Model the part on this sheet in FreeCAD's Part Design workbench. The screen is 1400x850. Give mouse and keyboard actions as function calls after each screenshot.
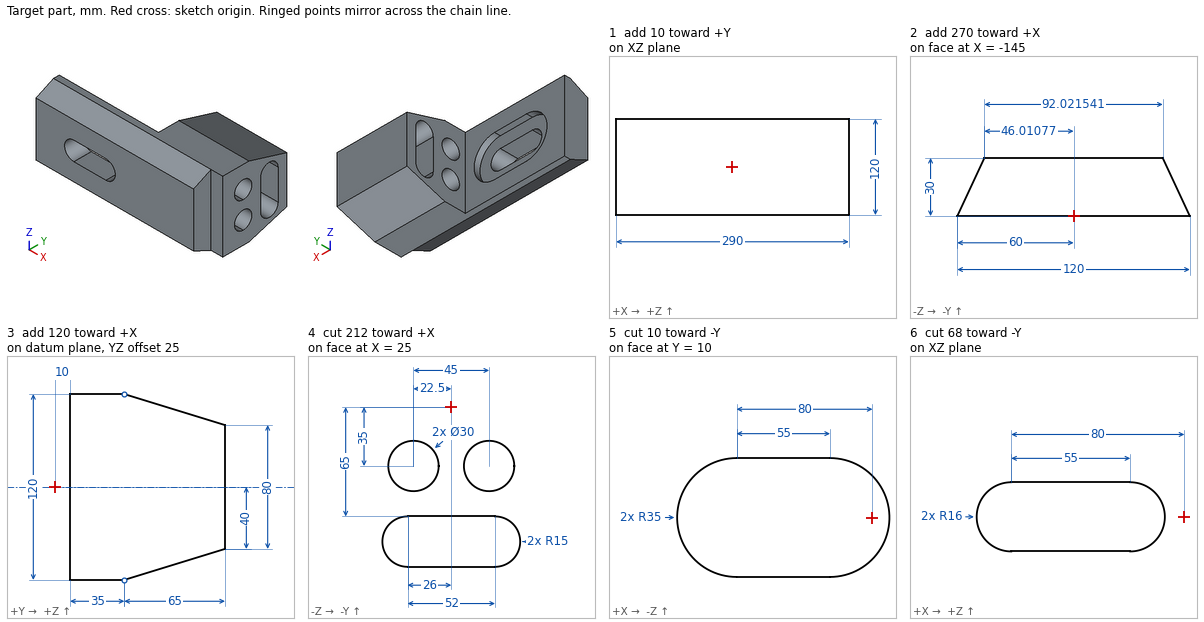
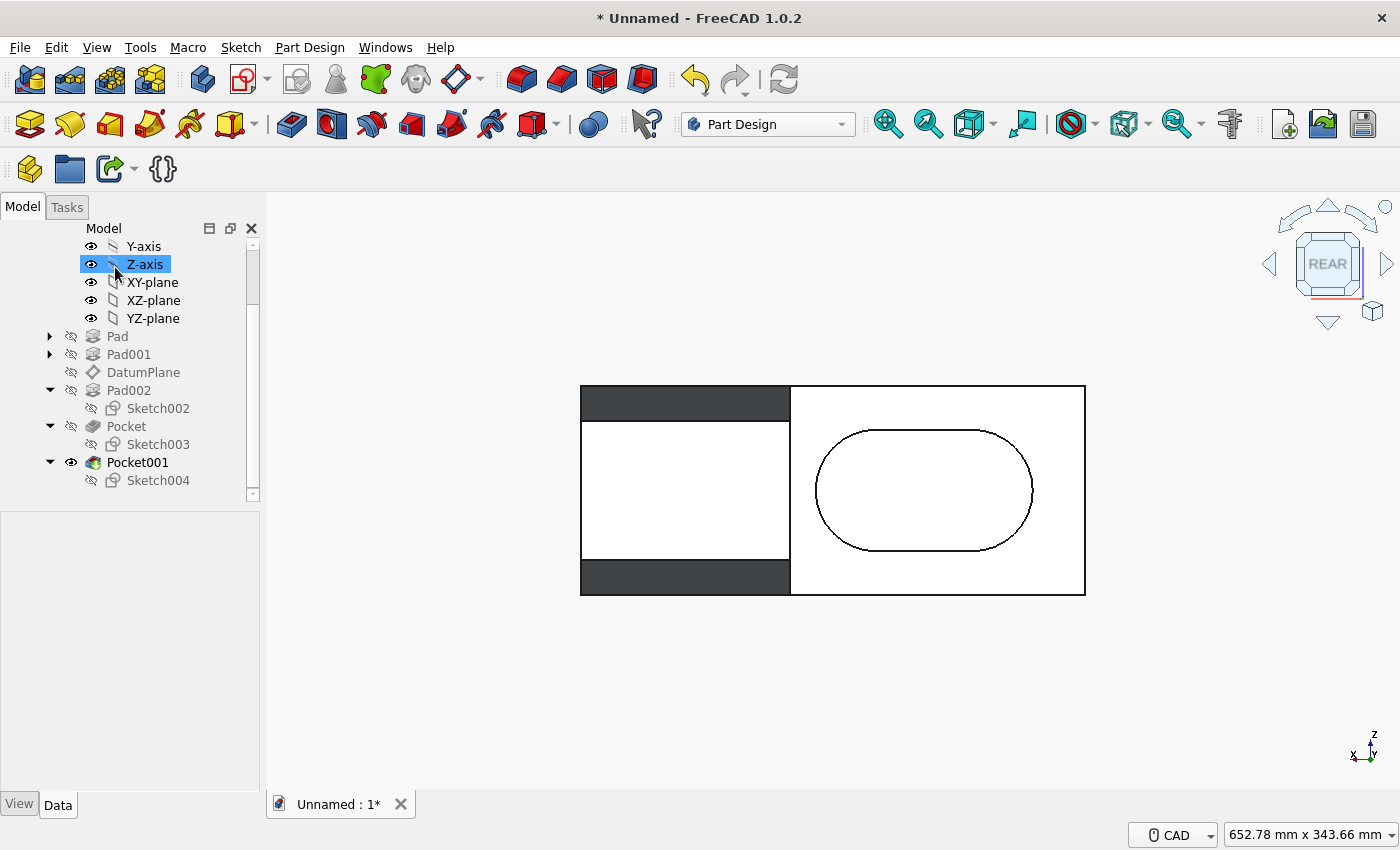
key(v)
key(f)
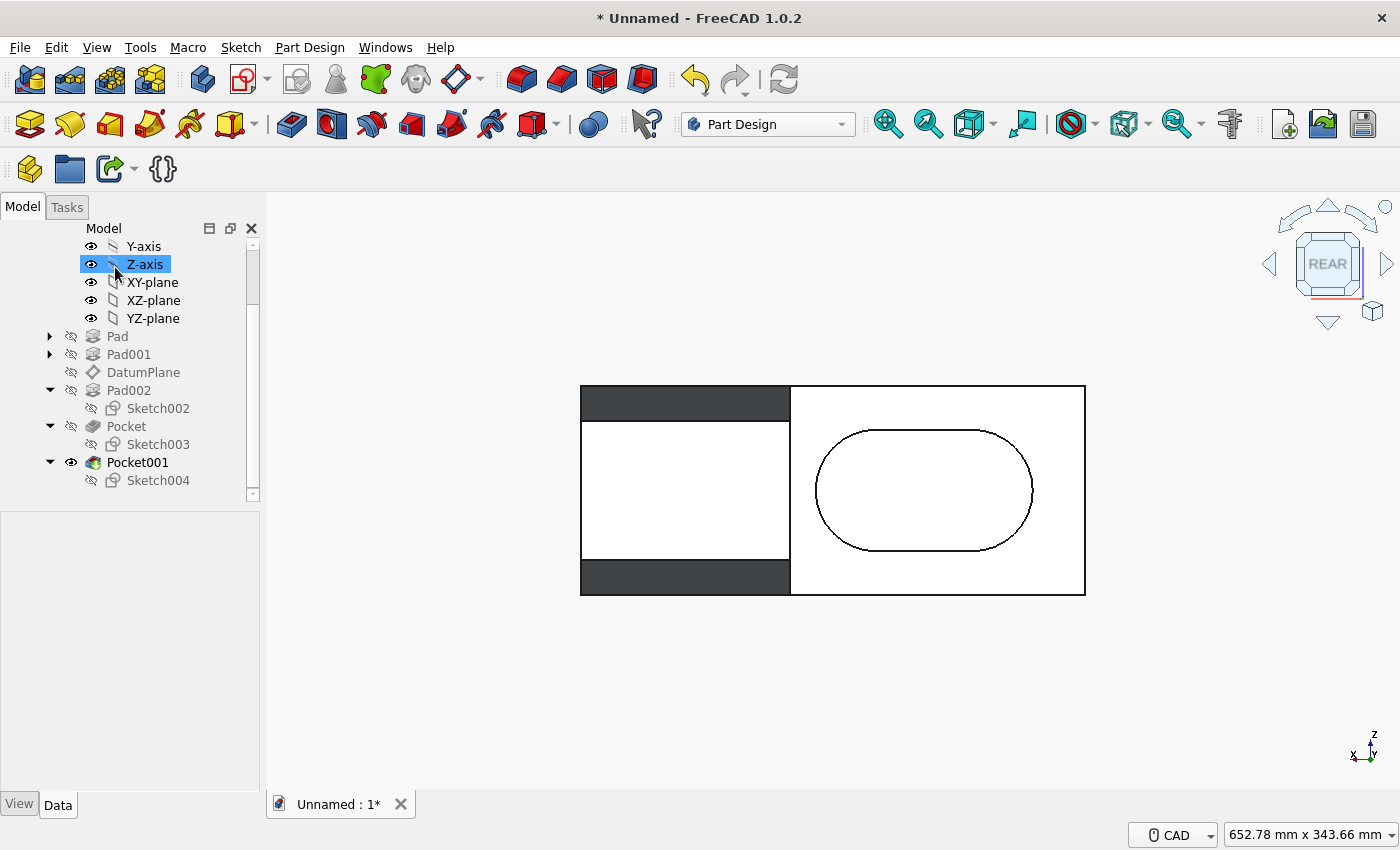
click(244, 80)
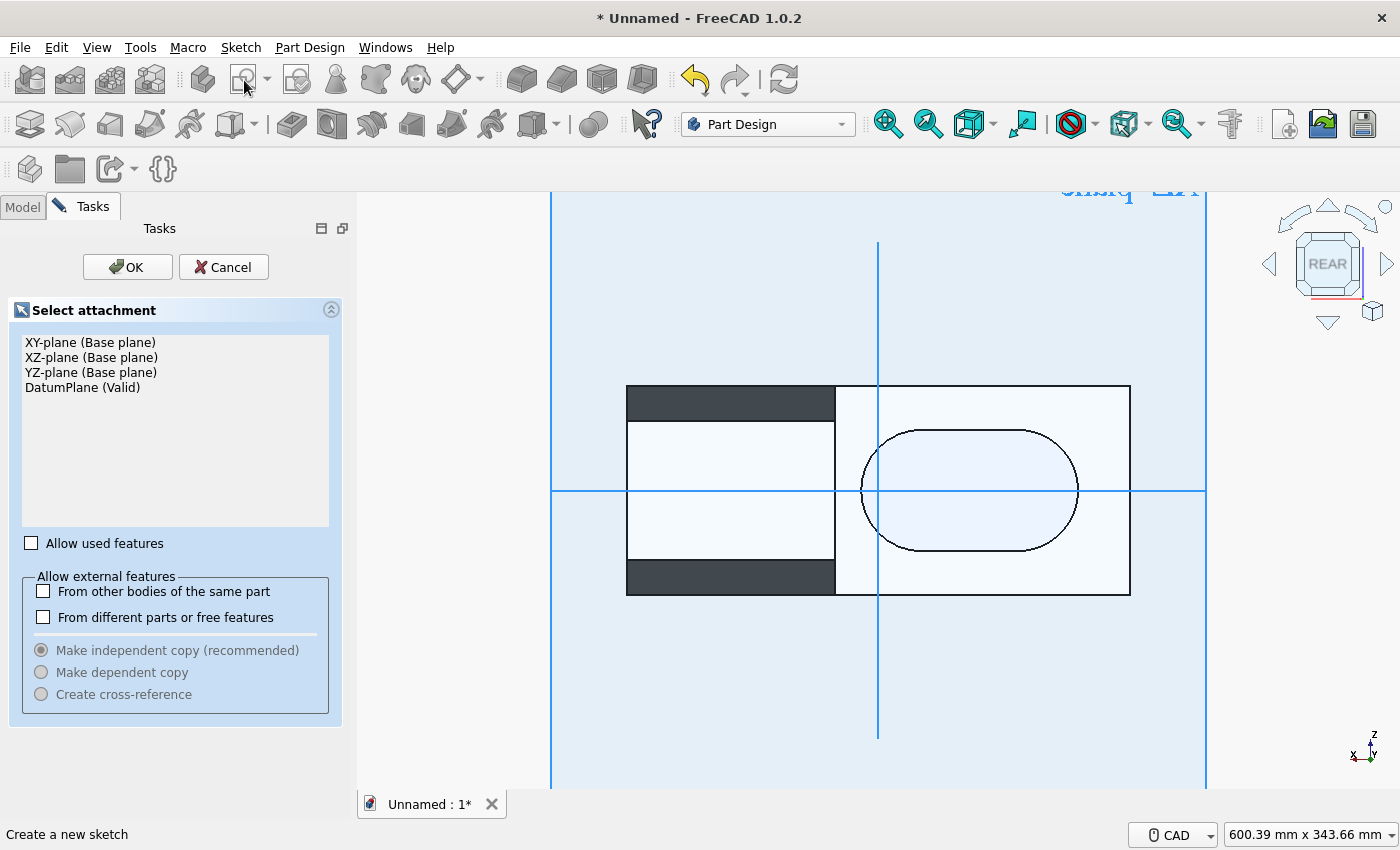
click(82, 358)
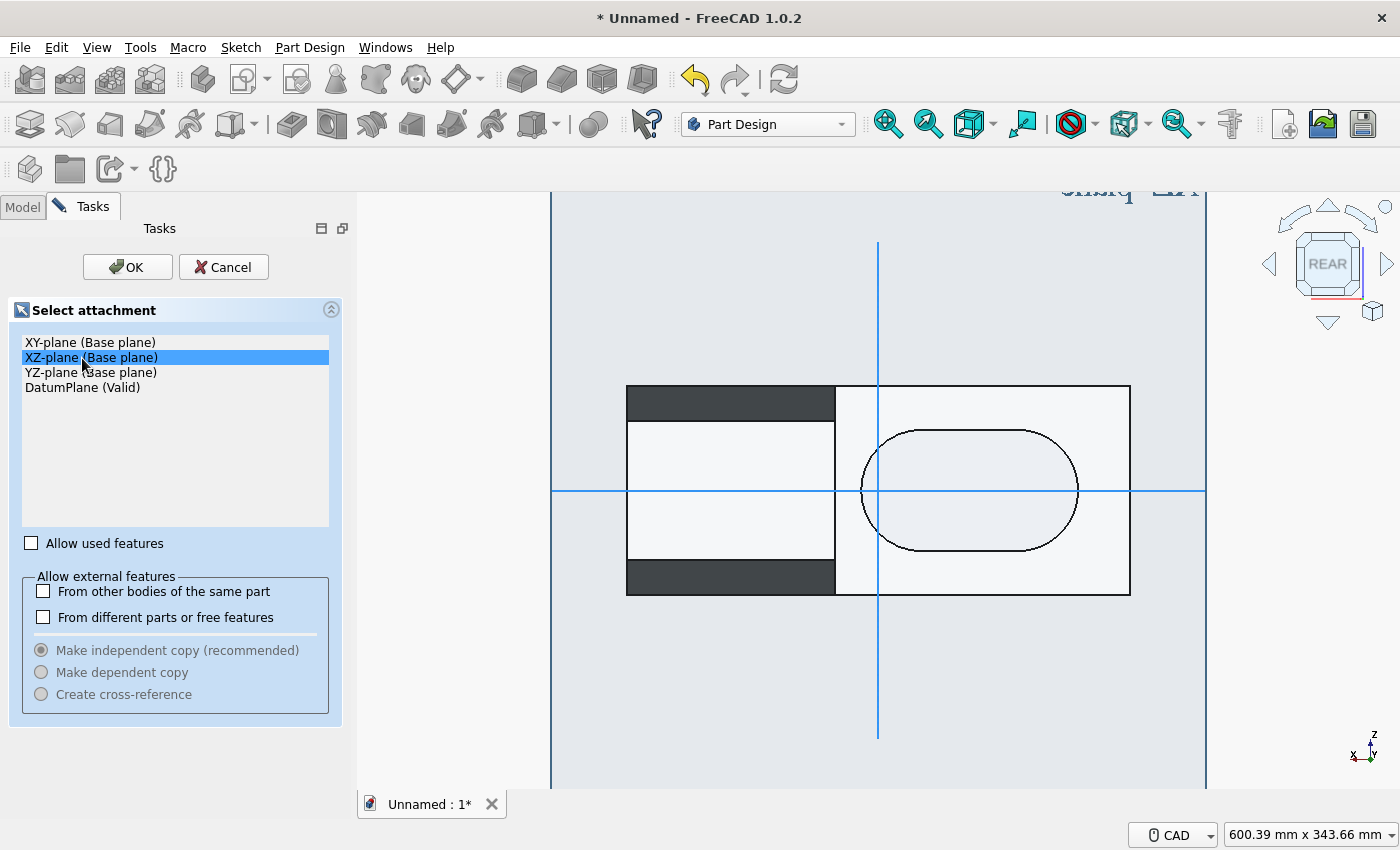
click(128, 267)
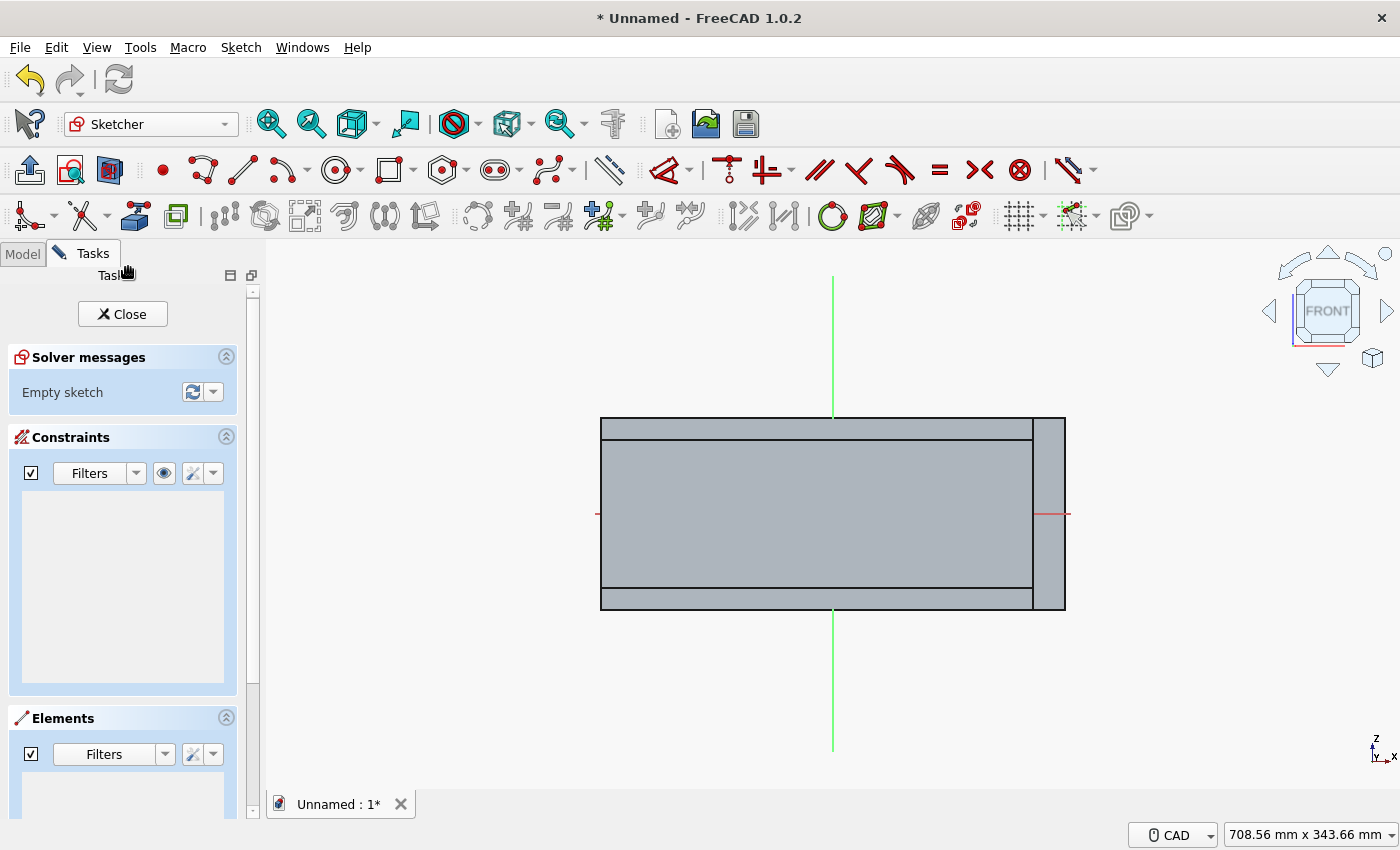
key(q)
key(s)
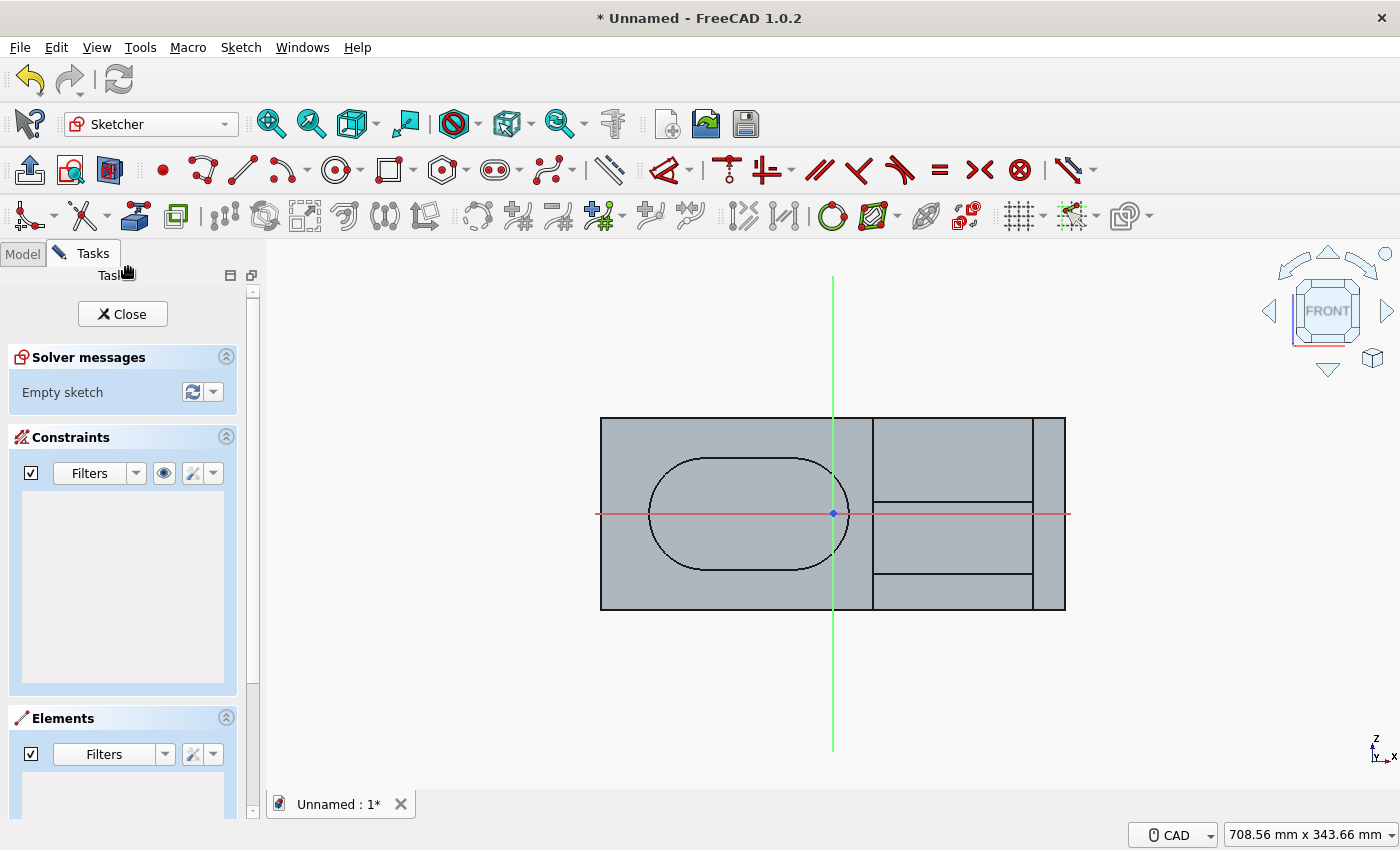
scroll(753, 514, up, 7)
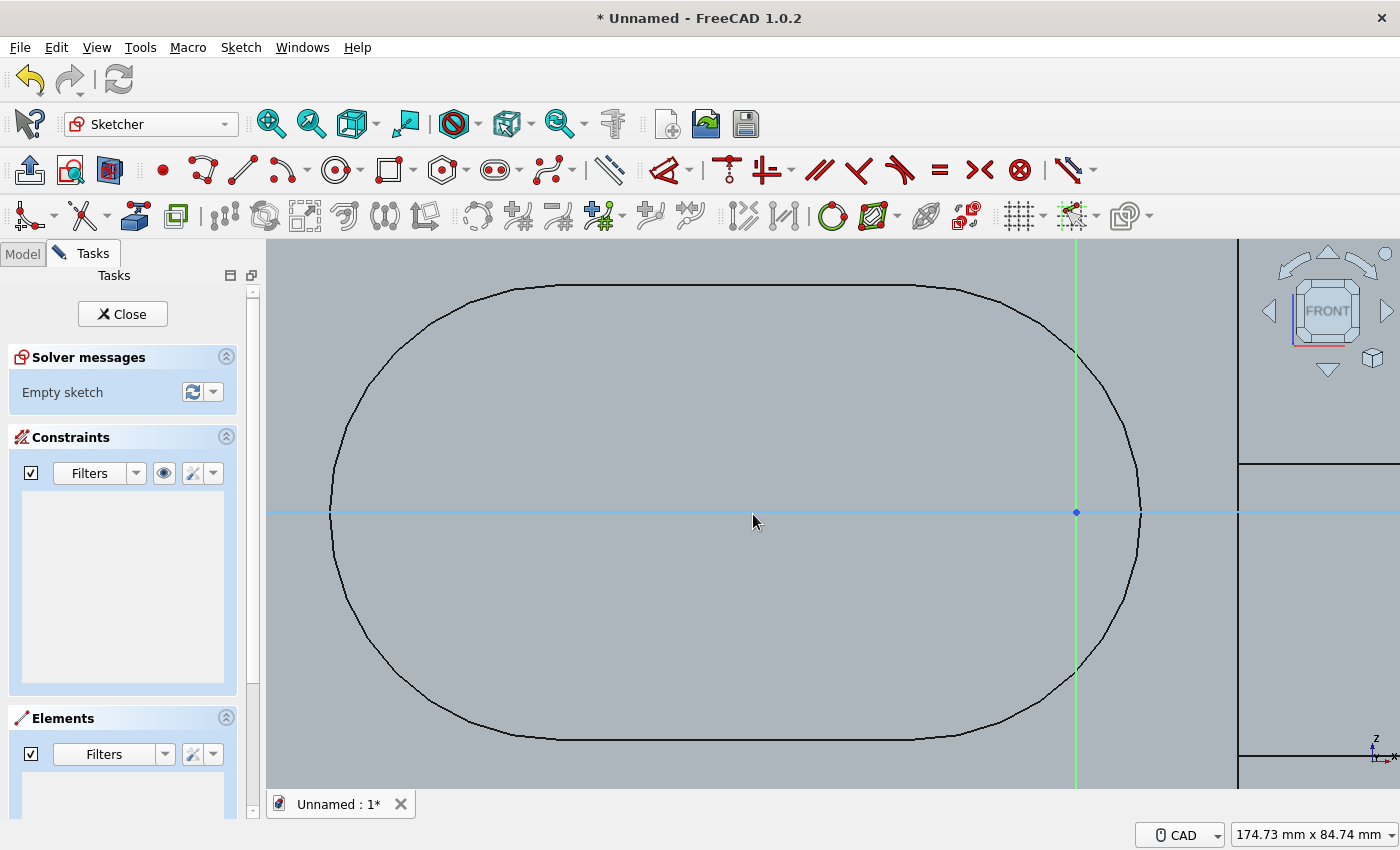
key(g)
key(s)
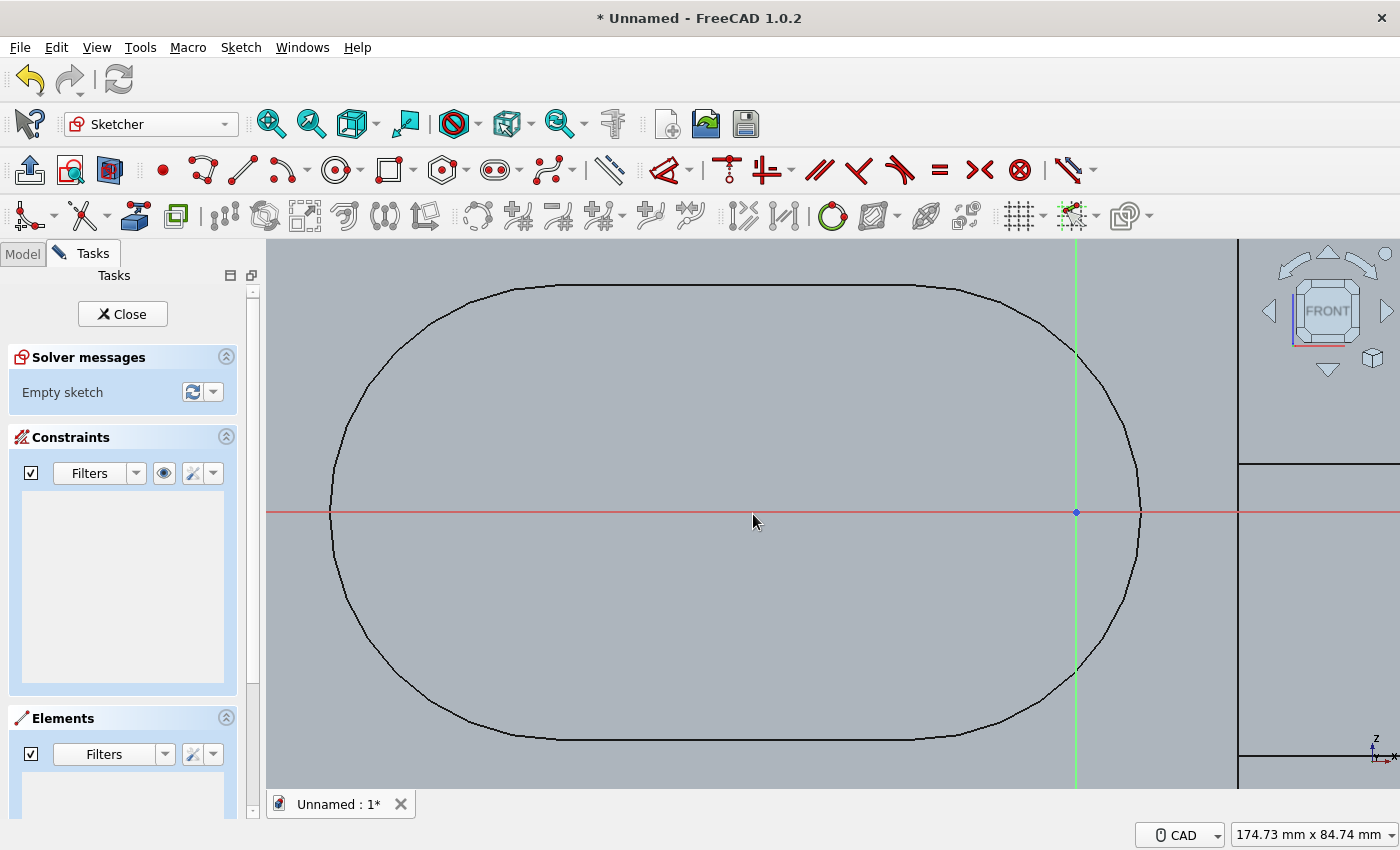
click(557, 512)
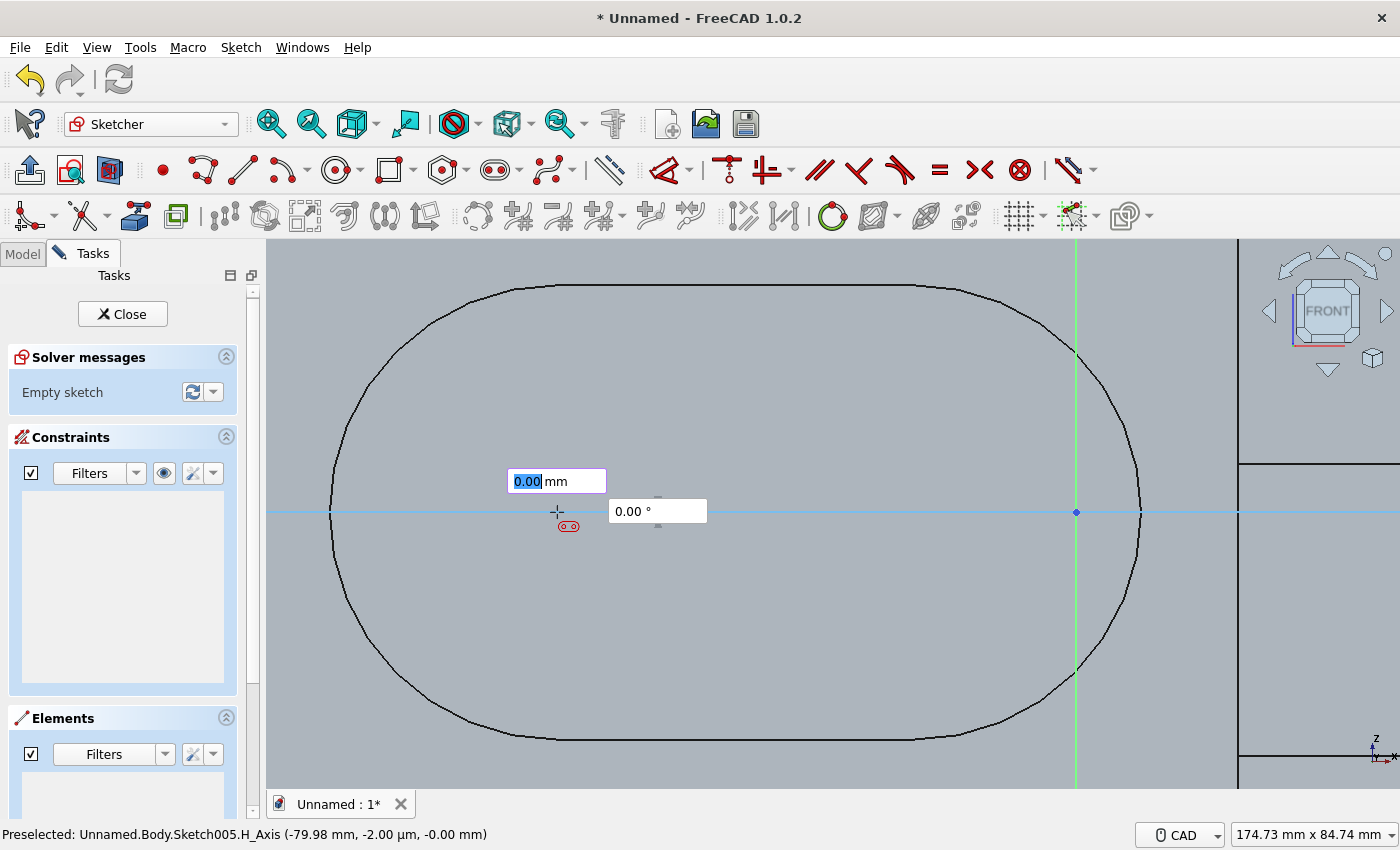
click(914, 503)